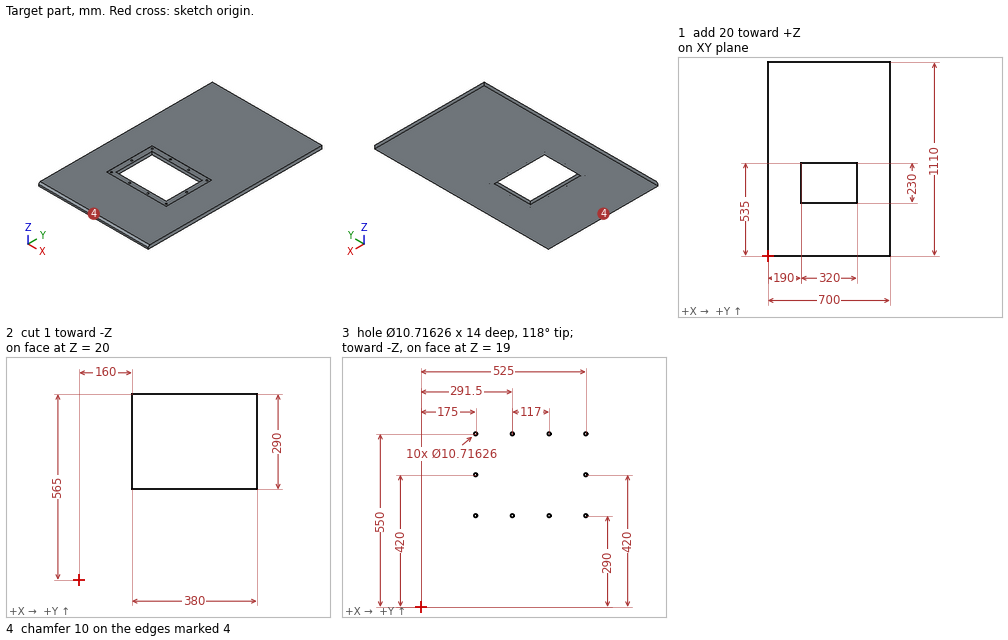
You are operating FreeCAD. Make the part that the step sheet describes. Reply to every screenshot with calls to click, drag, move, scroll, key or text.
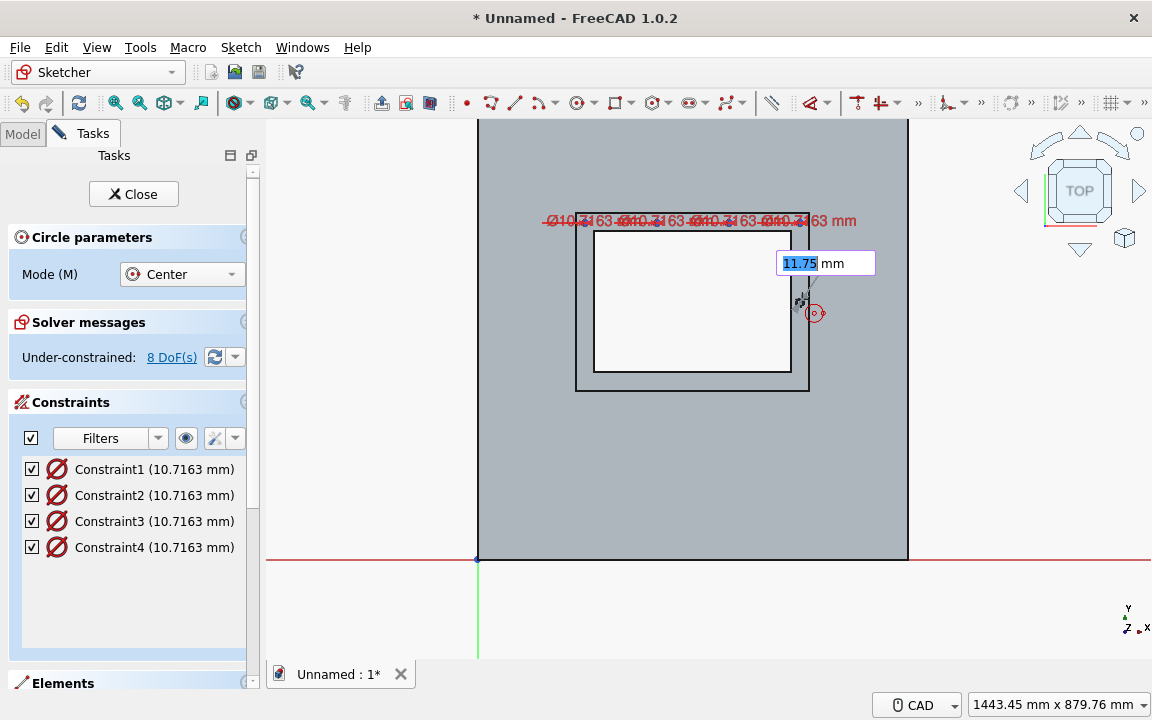
text(10.71626)
key(Return)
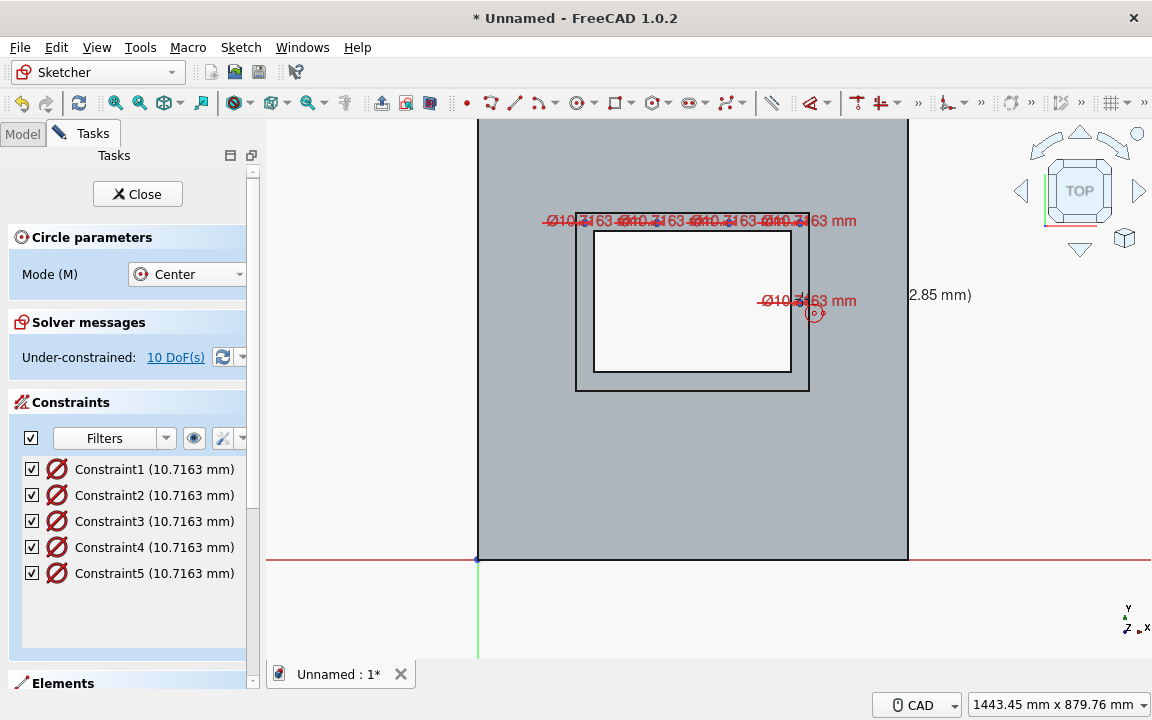
scroll(800, 382, up, 10)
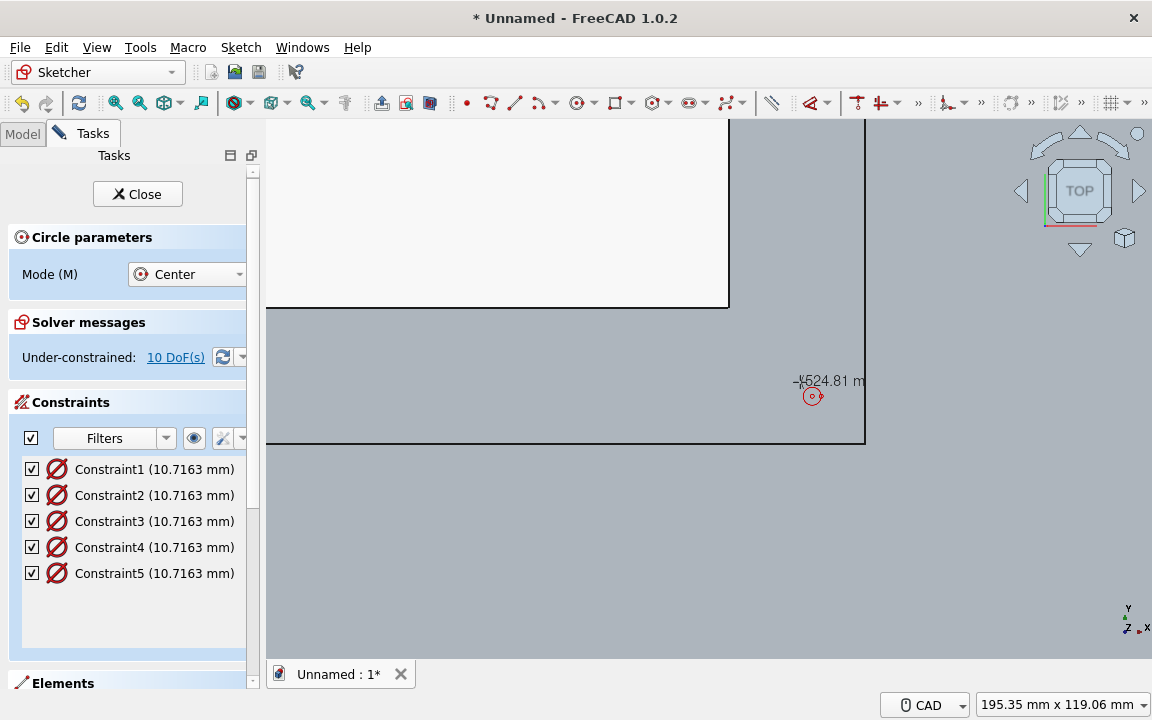
scroll(800, 382, down, 10)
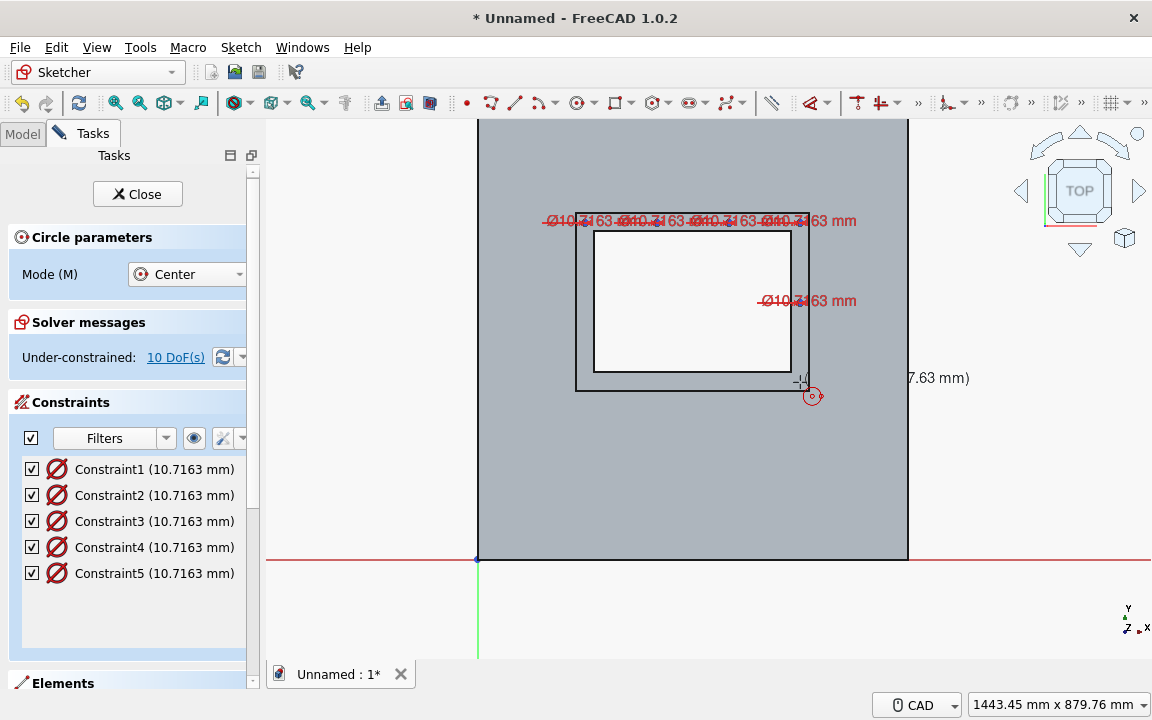
click(800, 382)
move(802, 379)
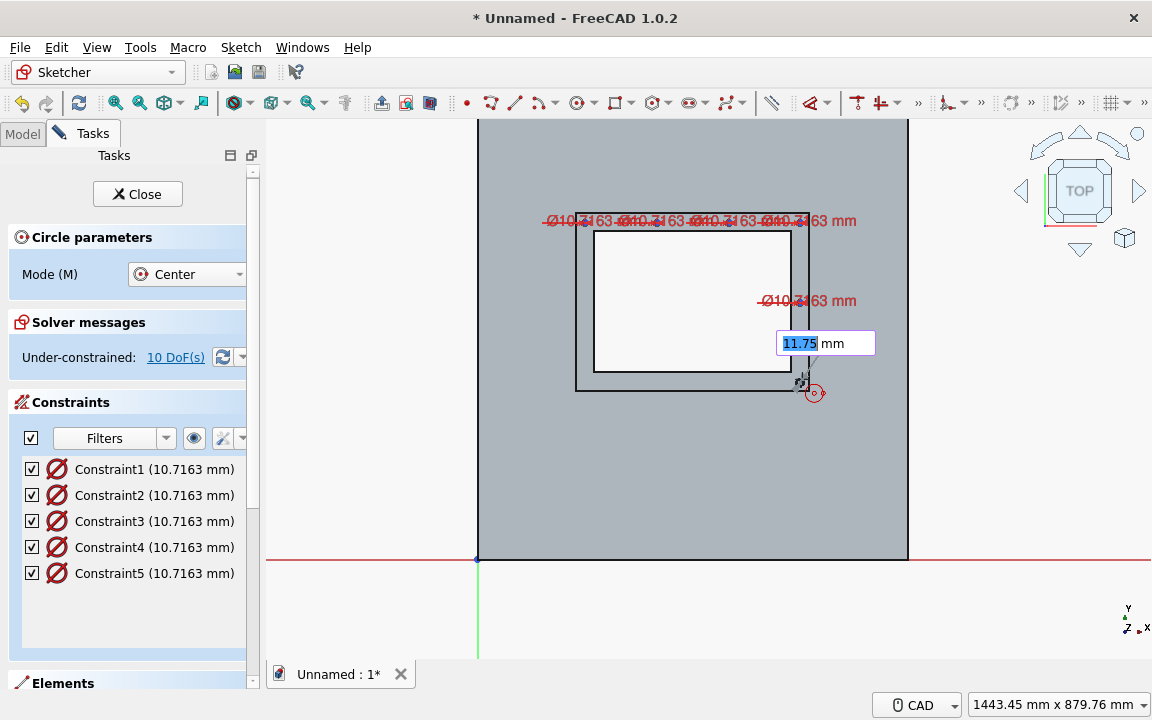
text(10.71626)
key(Return)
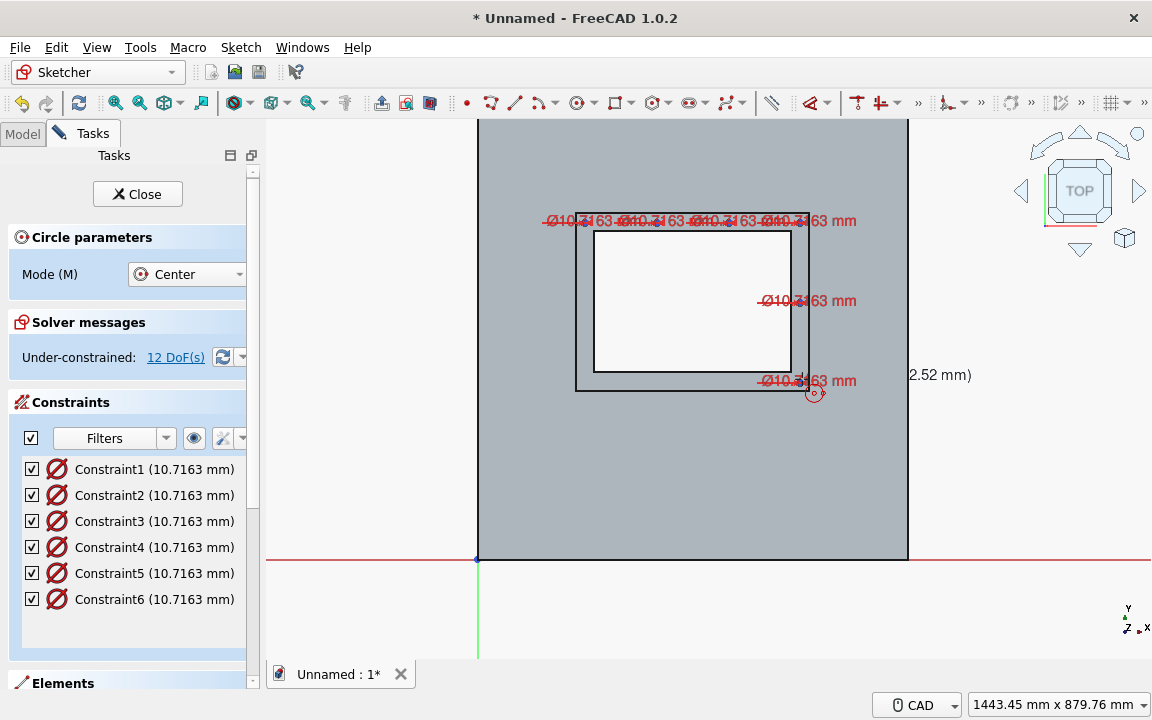
scroll(729, 382, up, 10)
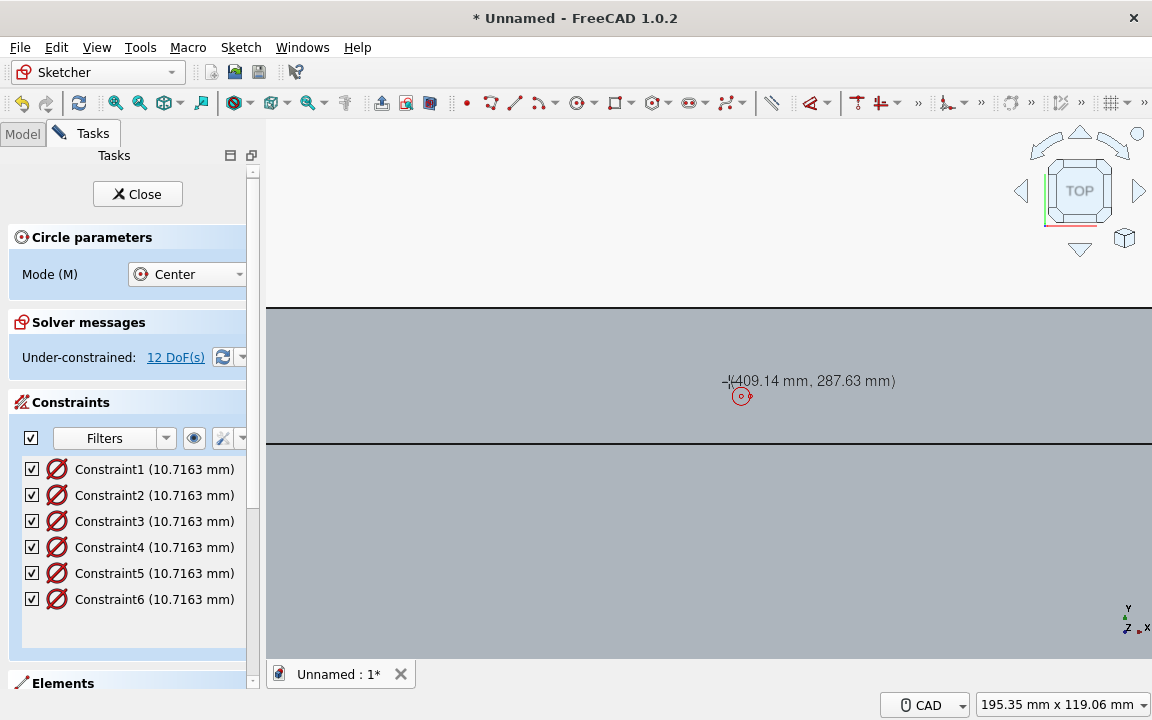
scroll(729, 382, down, 10)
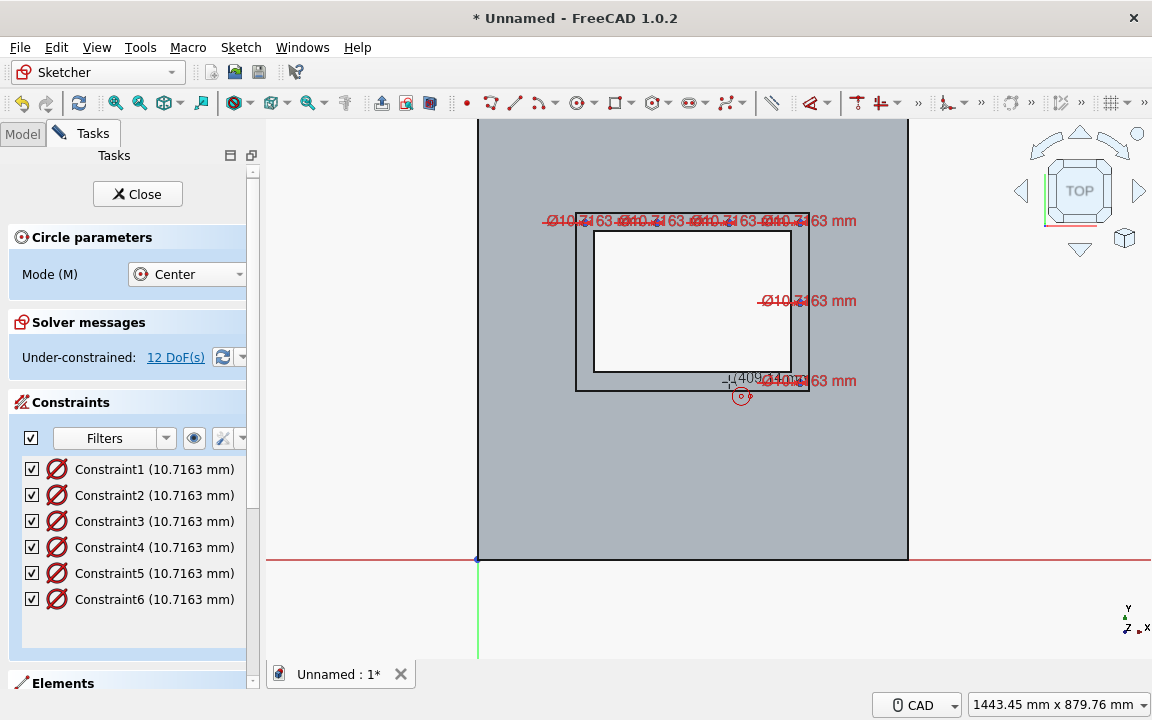
click(729, 382)
move(731, 379)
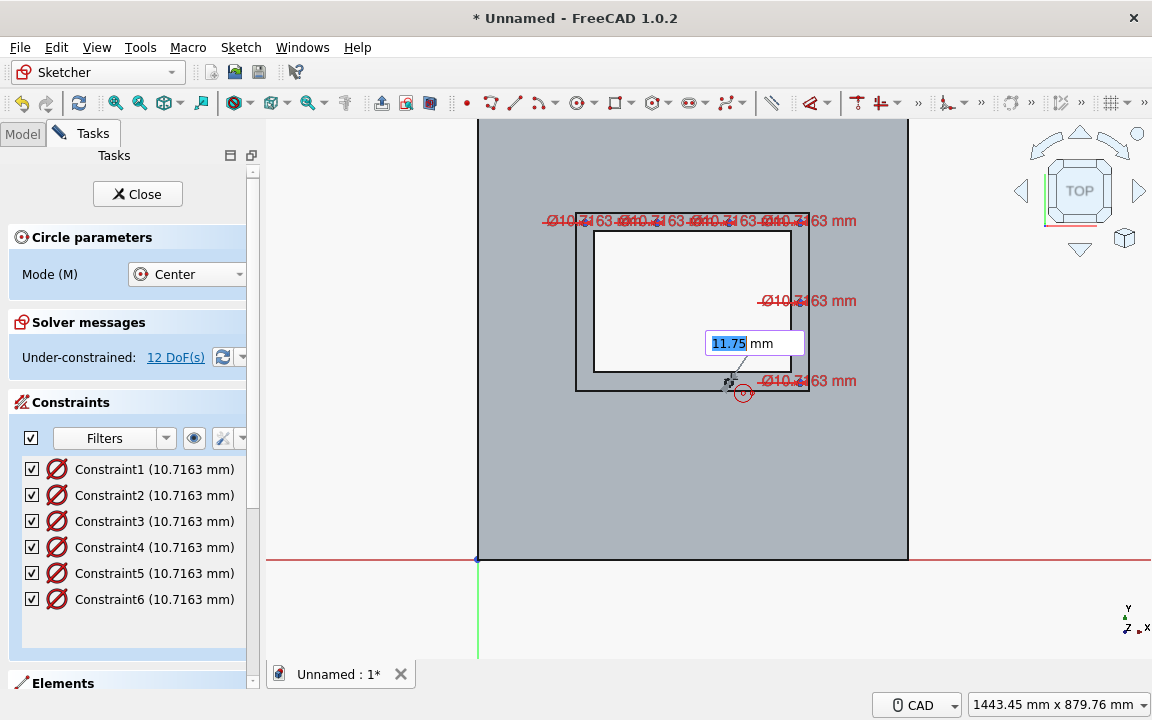
text(10.71626)
key(Return)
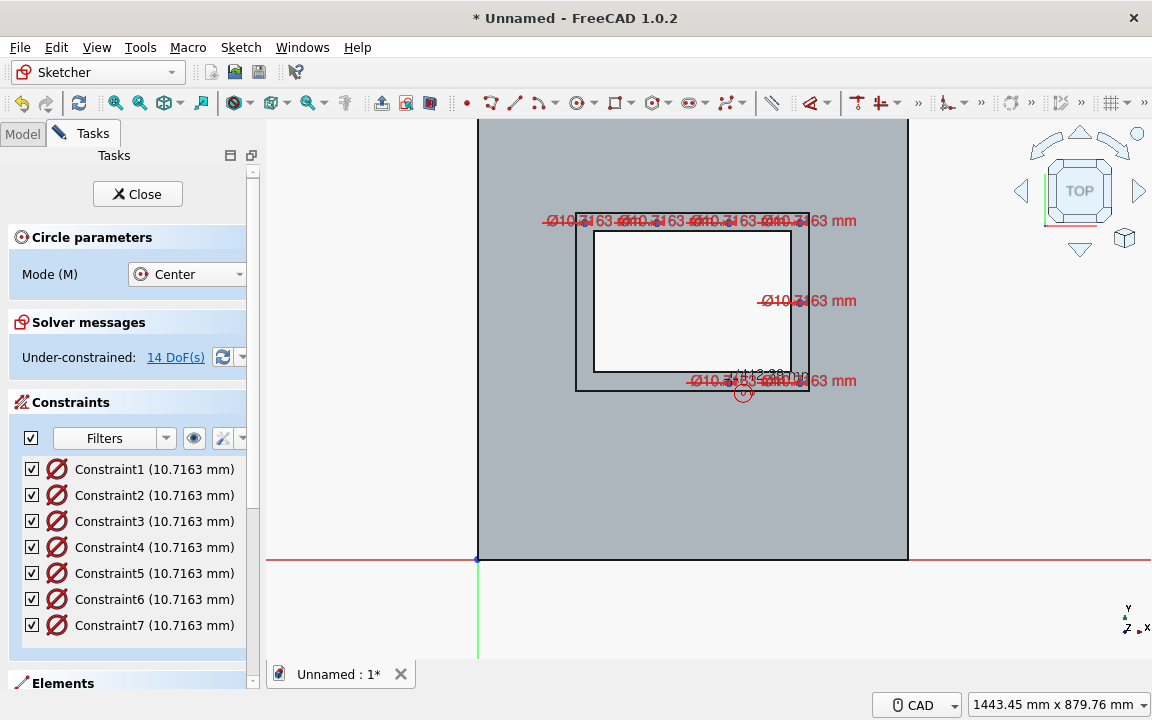
scroll(657, 382, up, 10)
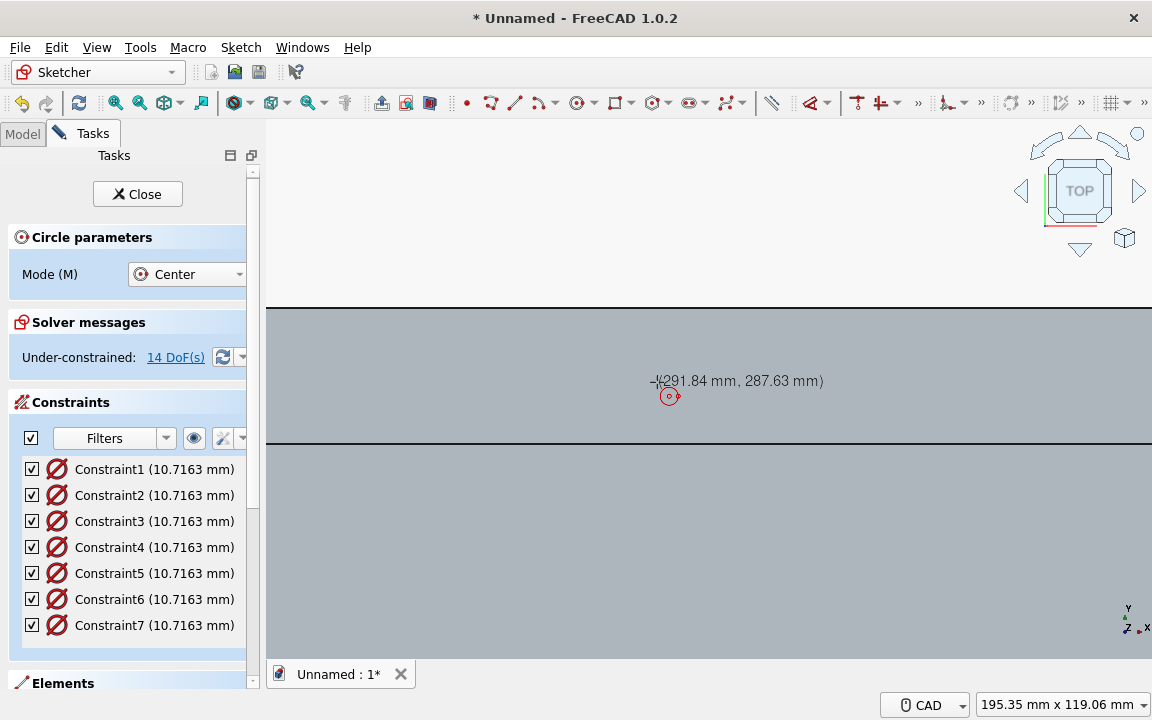
scroll(657, 382, down, 10)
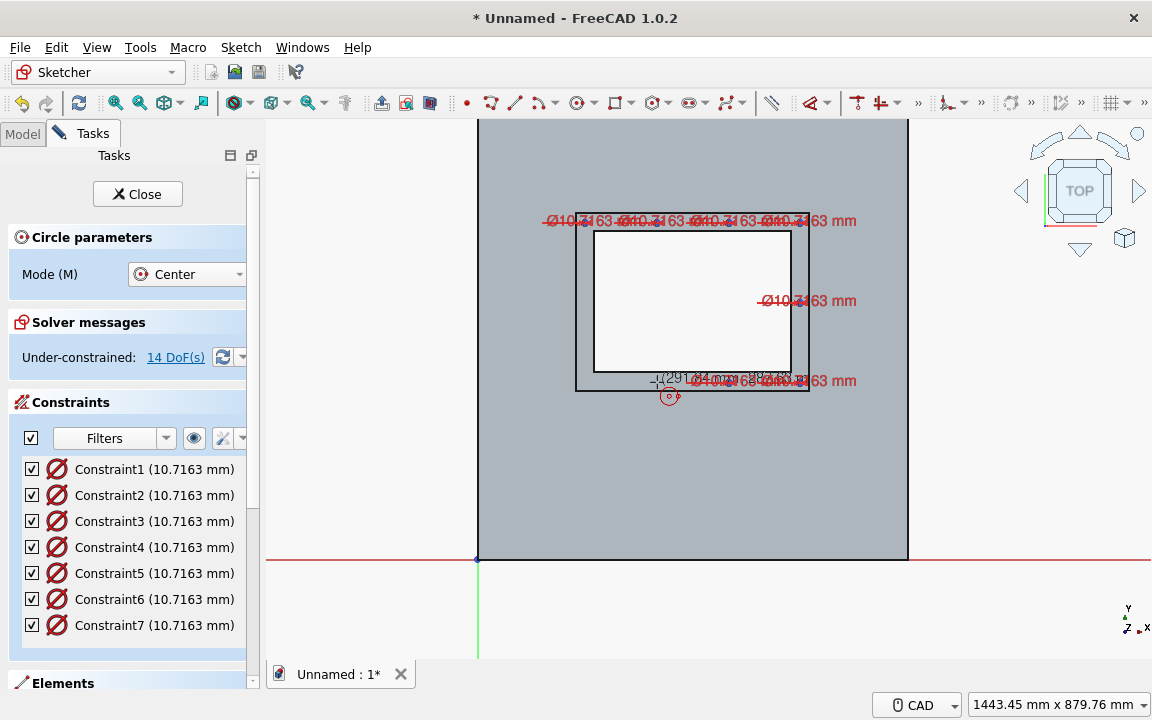
click(657, 382)
move(659, 379)